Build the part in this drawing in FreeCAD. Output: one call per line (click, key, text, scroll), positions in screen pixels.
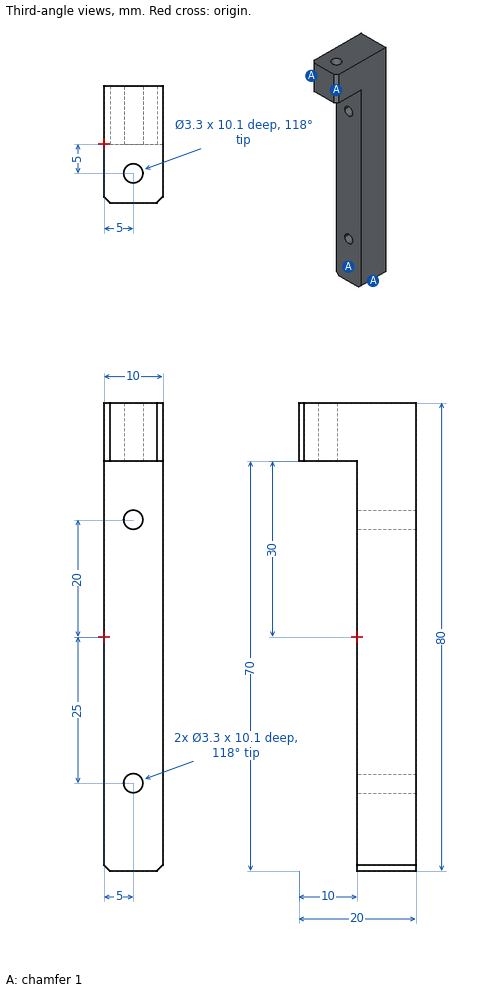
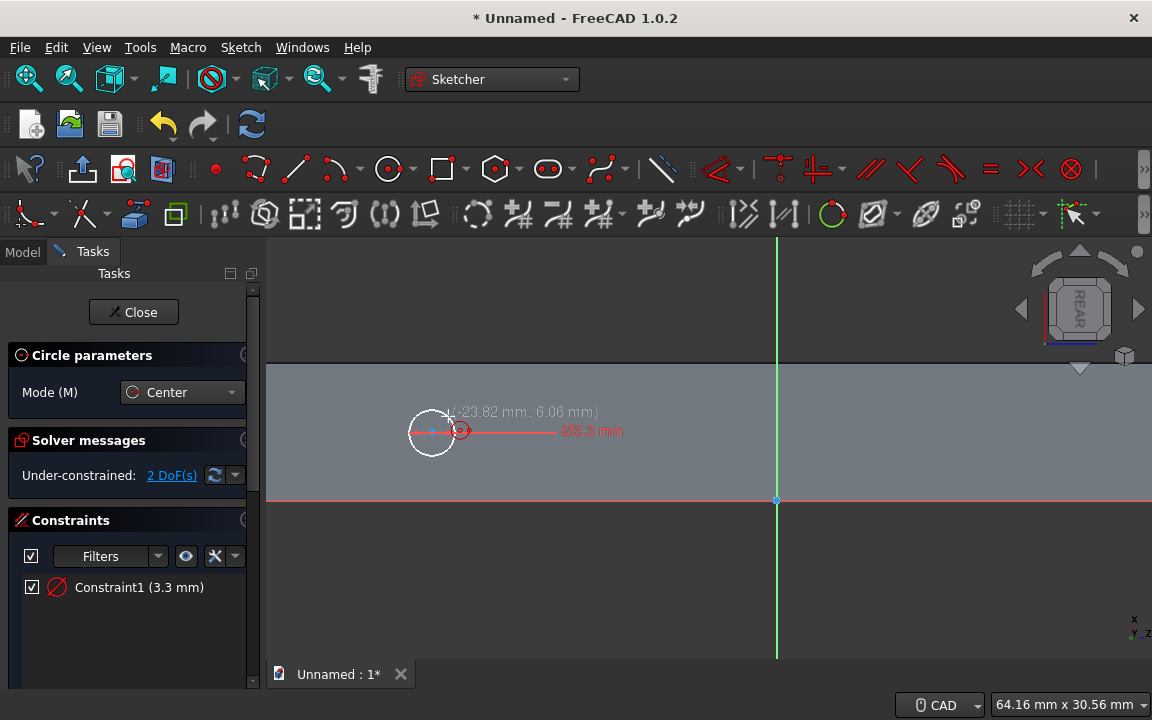
scroll(433, 434, down, 2)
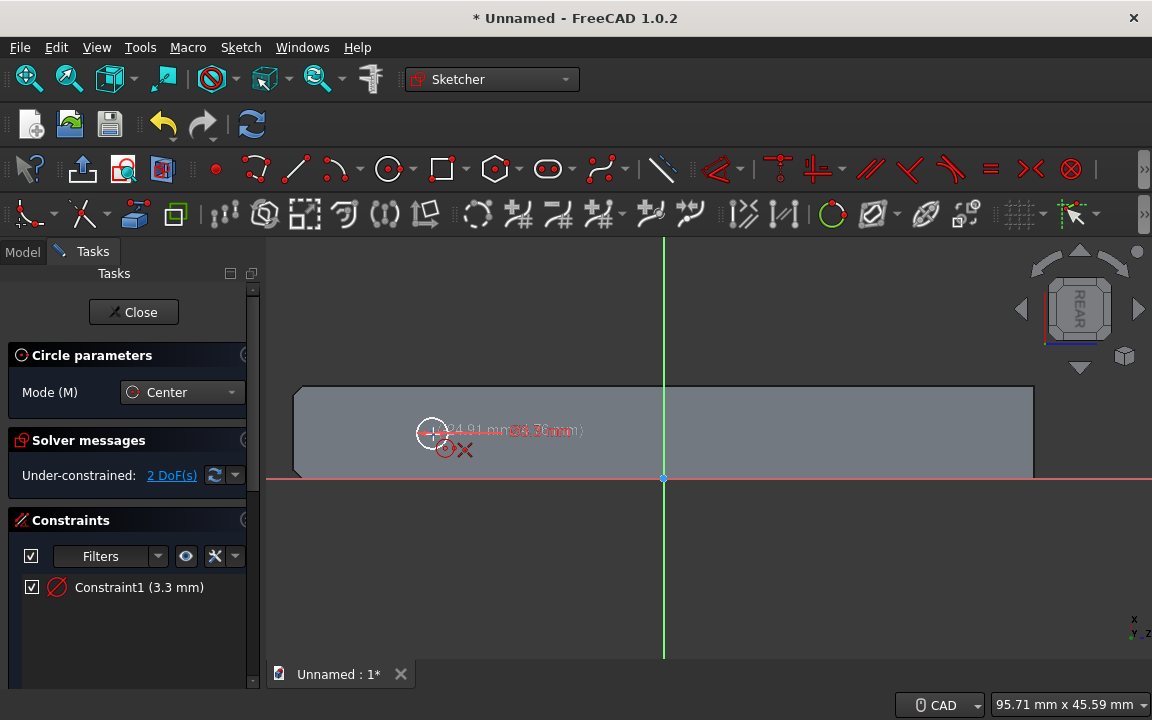
scroll(849, 433, up, 2)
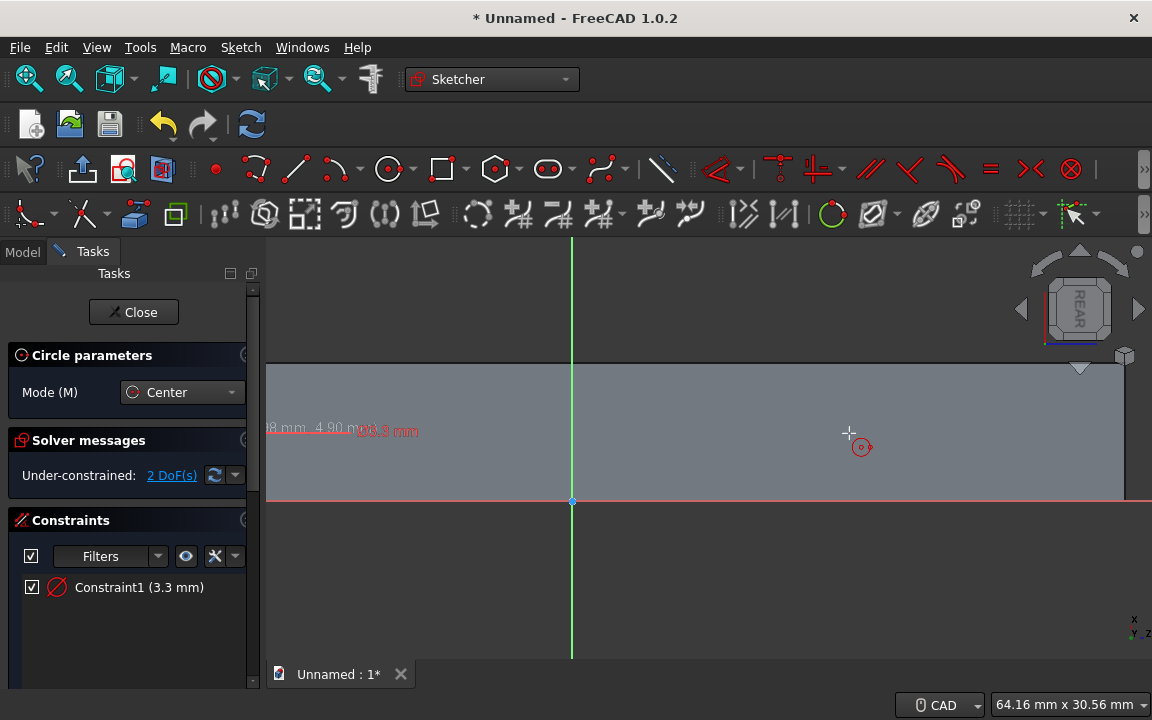
click(848, 432)
move(864, 416)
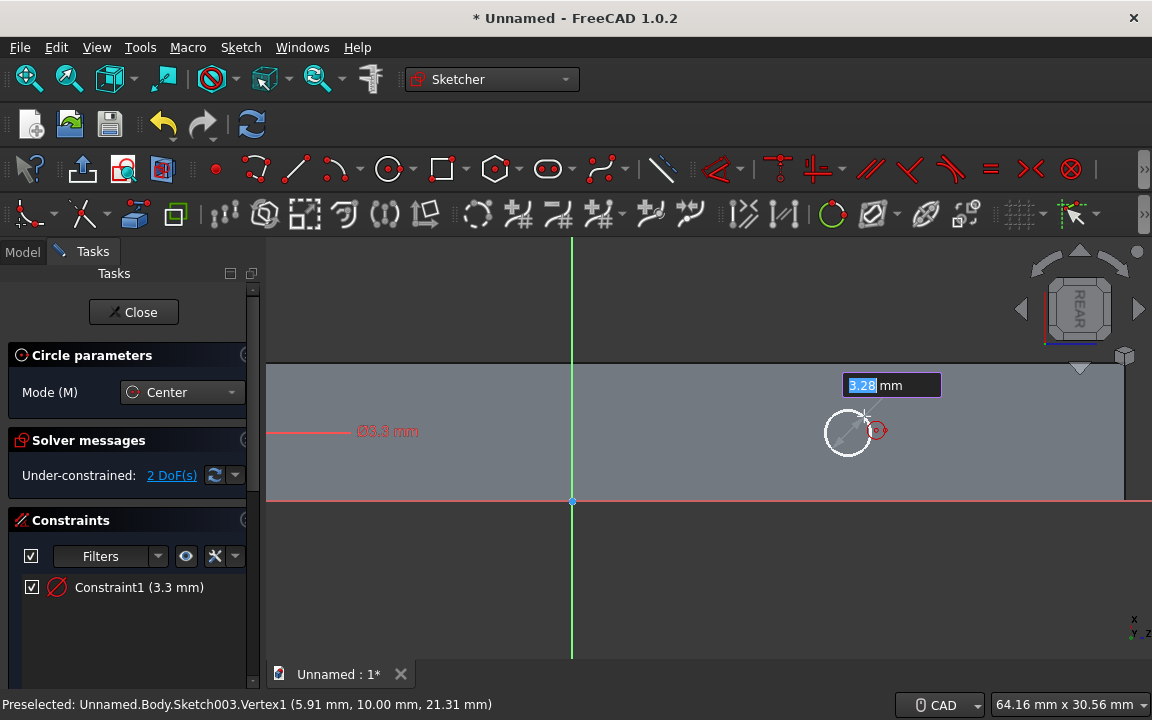
text(3.3)
key(Return)
key(Escape)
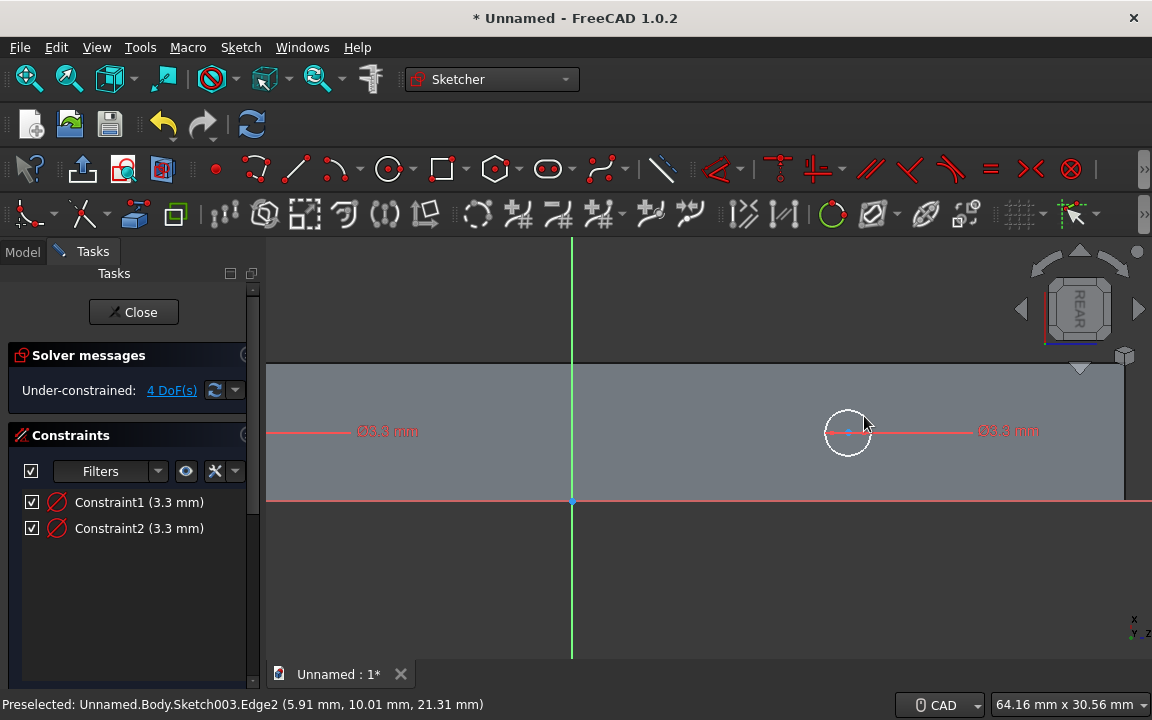
scroll(850, 433, down, 2)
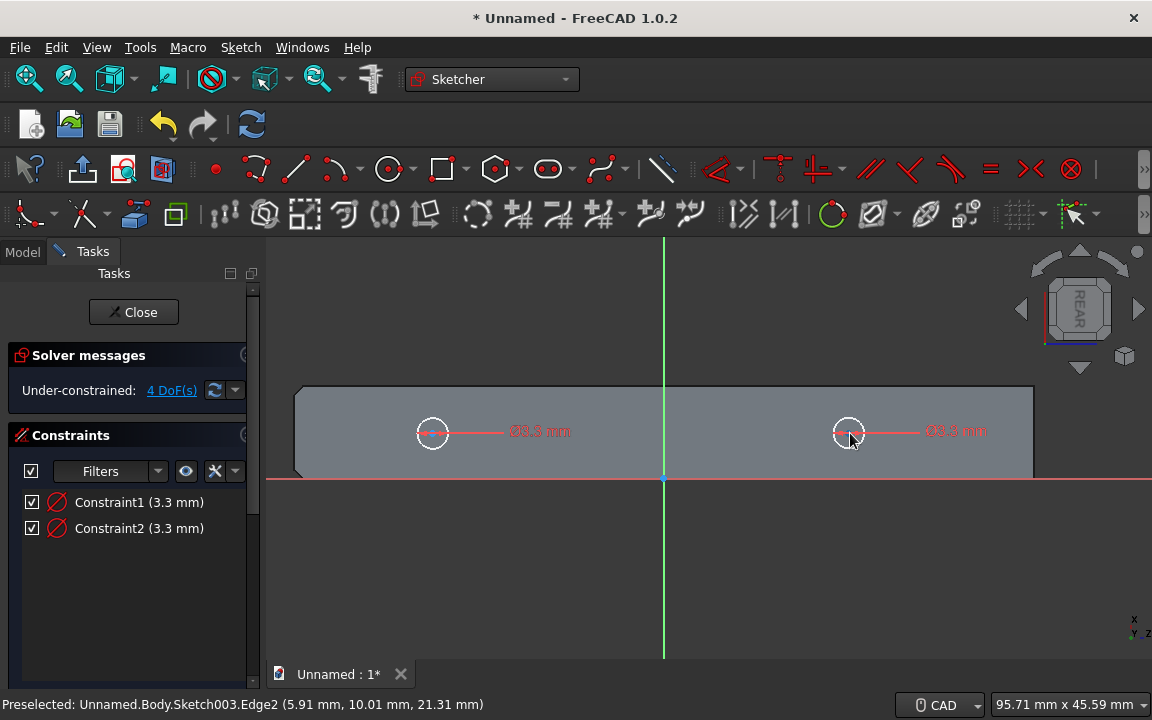
click(433, 433)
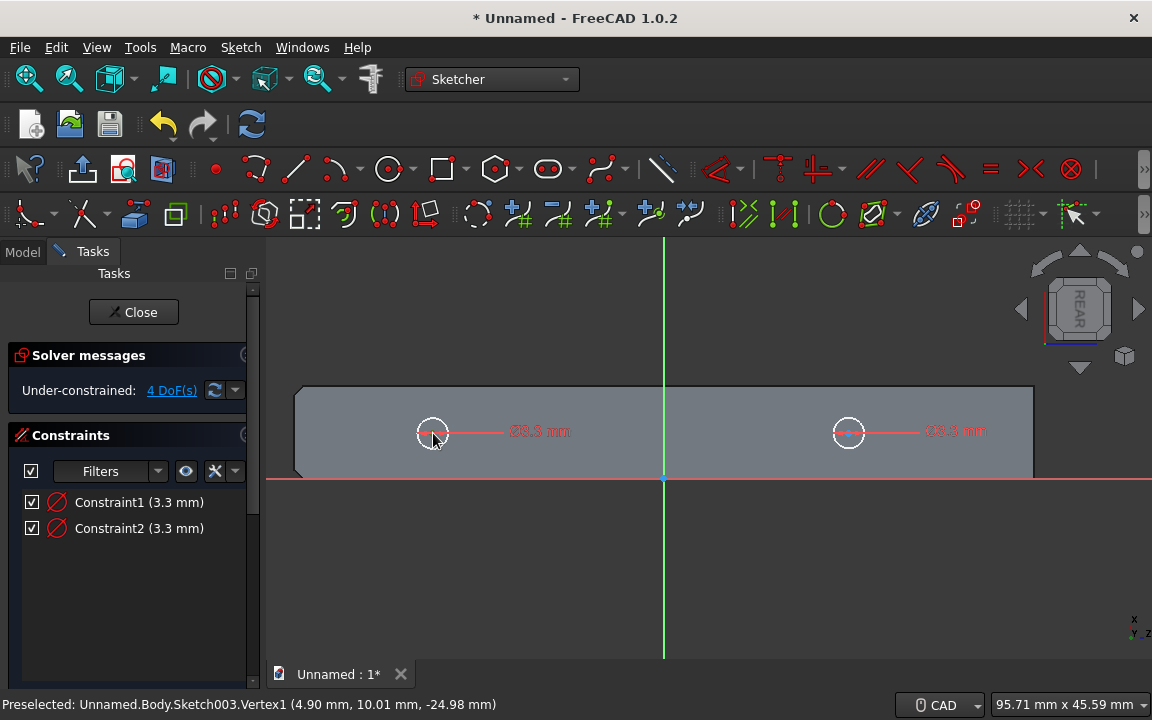
click(849, 433)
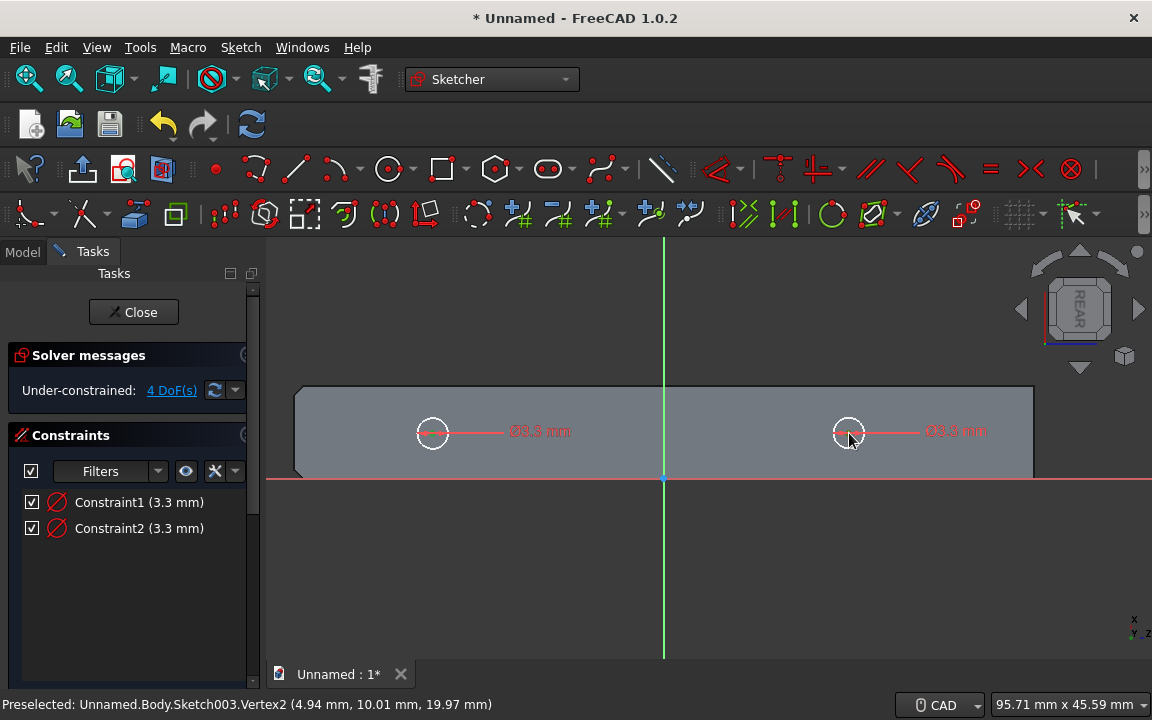
key(h)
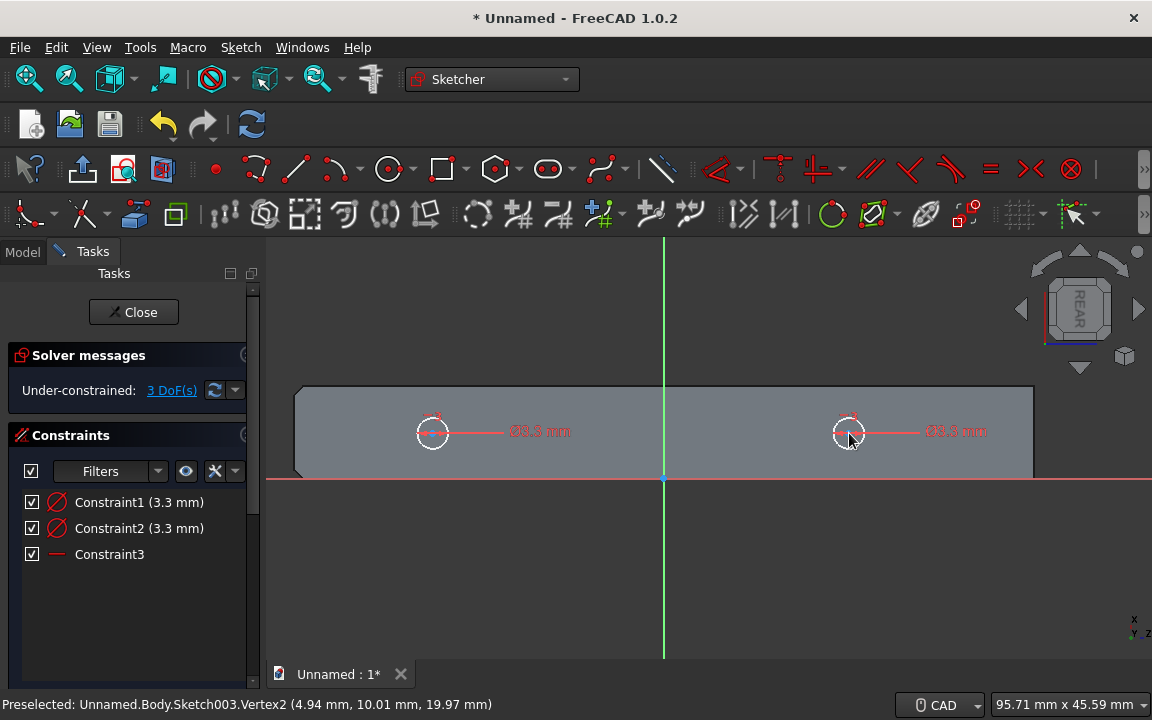
click(433, 433)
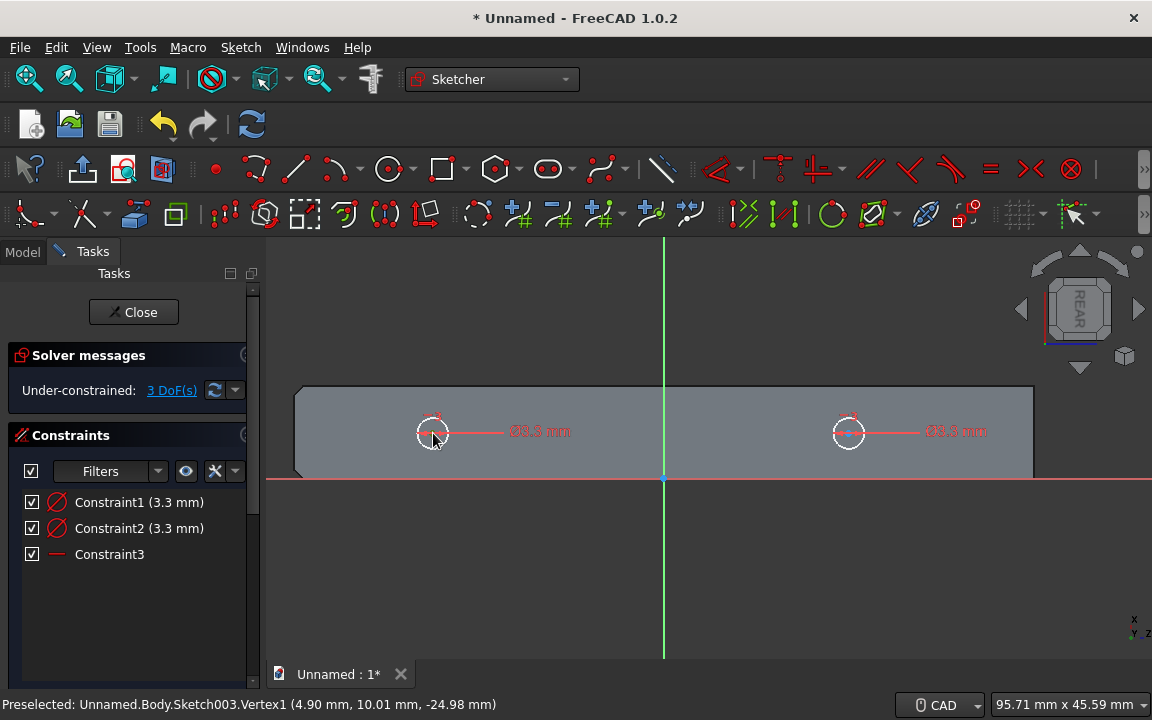
key(i)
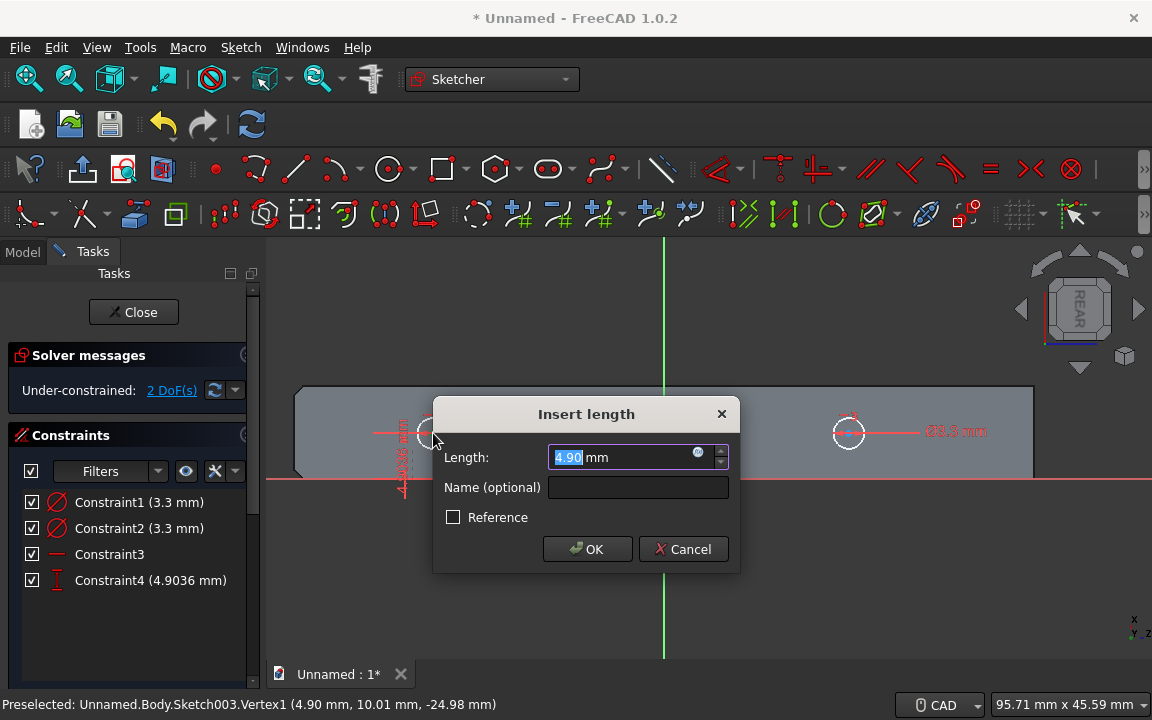
text(5)
key(Return)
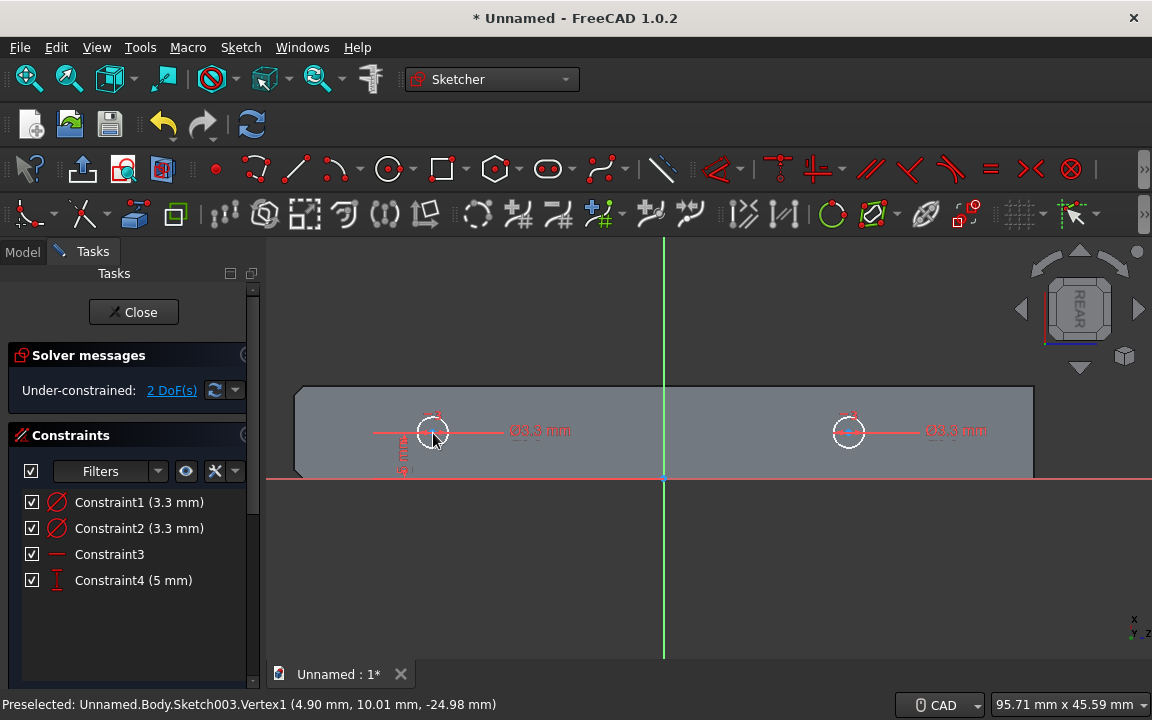
click(433, 433)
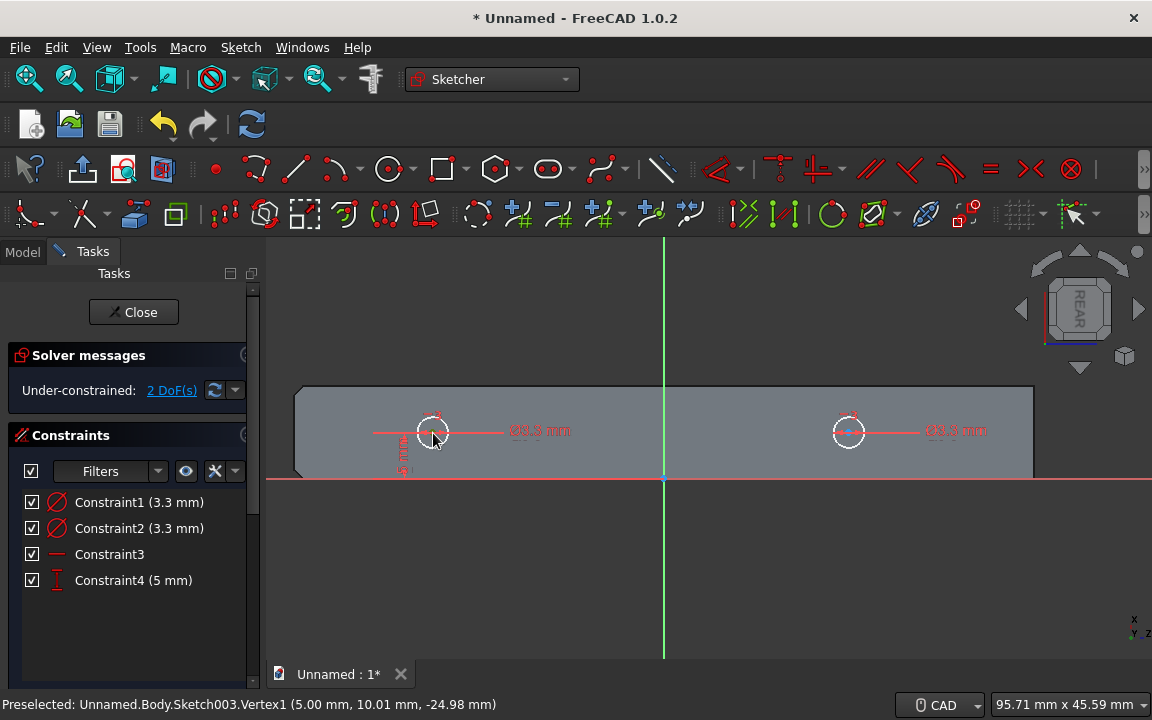
key(l)